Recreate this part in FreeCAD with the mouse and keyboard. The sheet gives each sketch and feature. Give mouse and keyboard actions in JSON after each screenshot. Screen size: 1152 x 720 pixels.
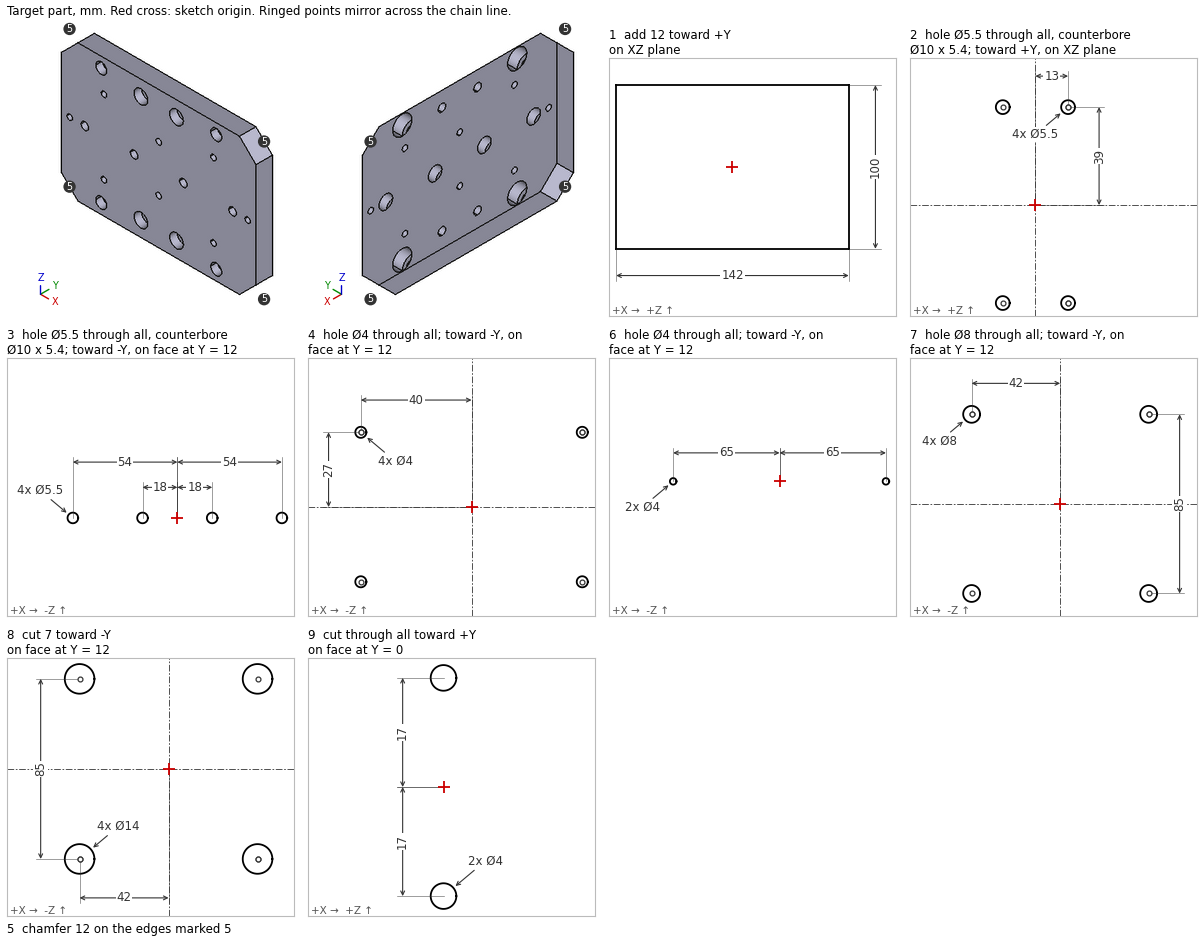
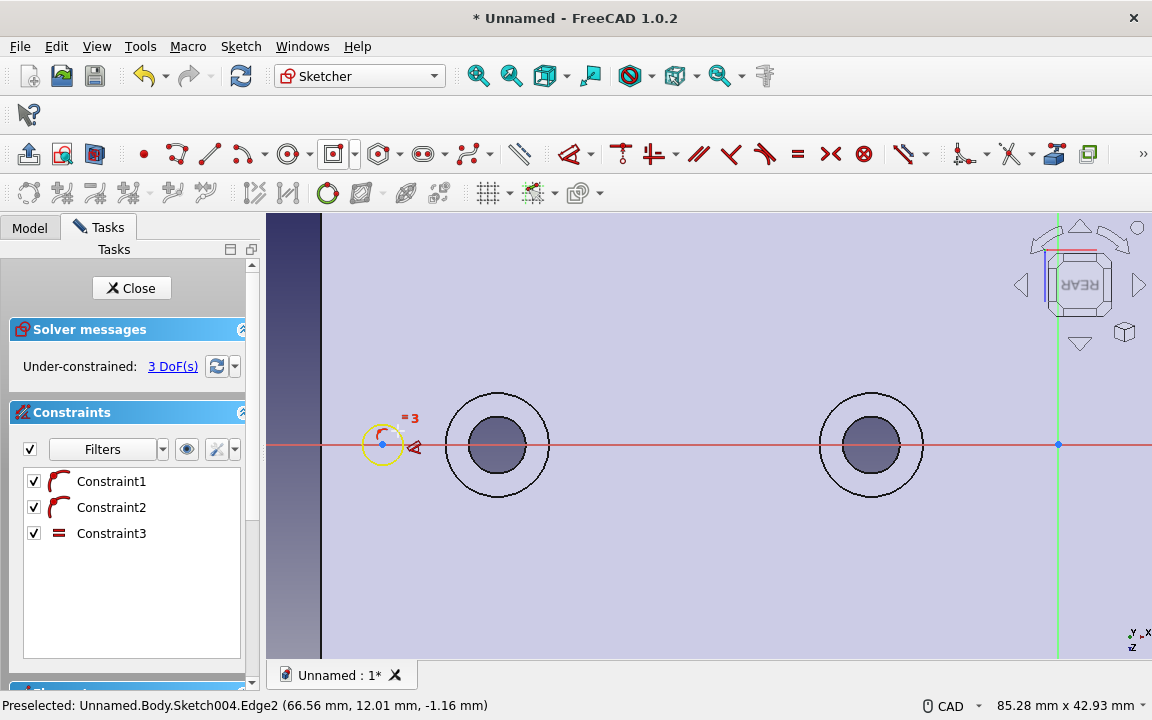
{"action": "left_click", "coordinate": [397, 431]}
{"action": "left_click", "coordinate": [420, 409]}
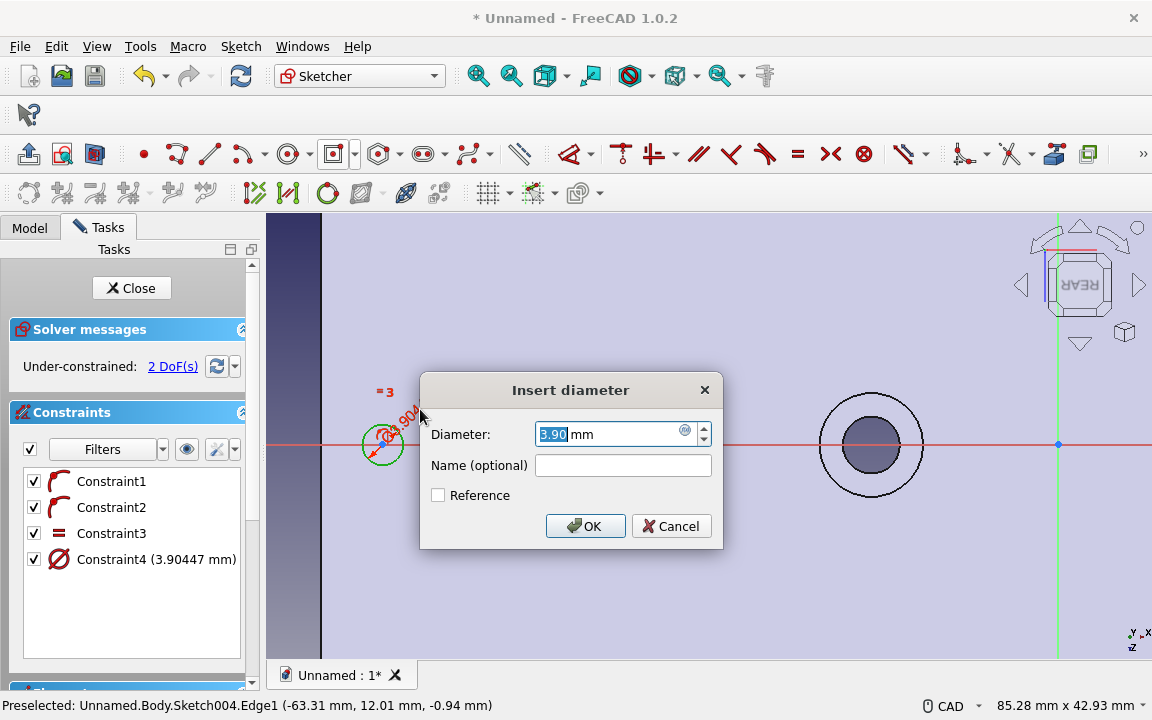
{"action": "type", "text": "4"}
{"action": "key", "text": "Return"}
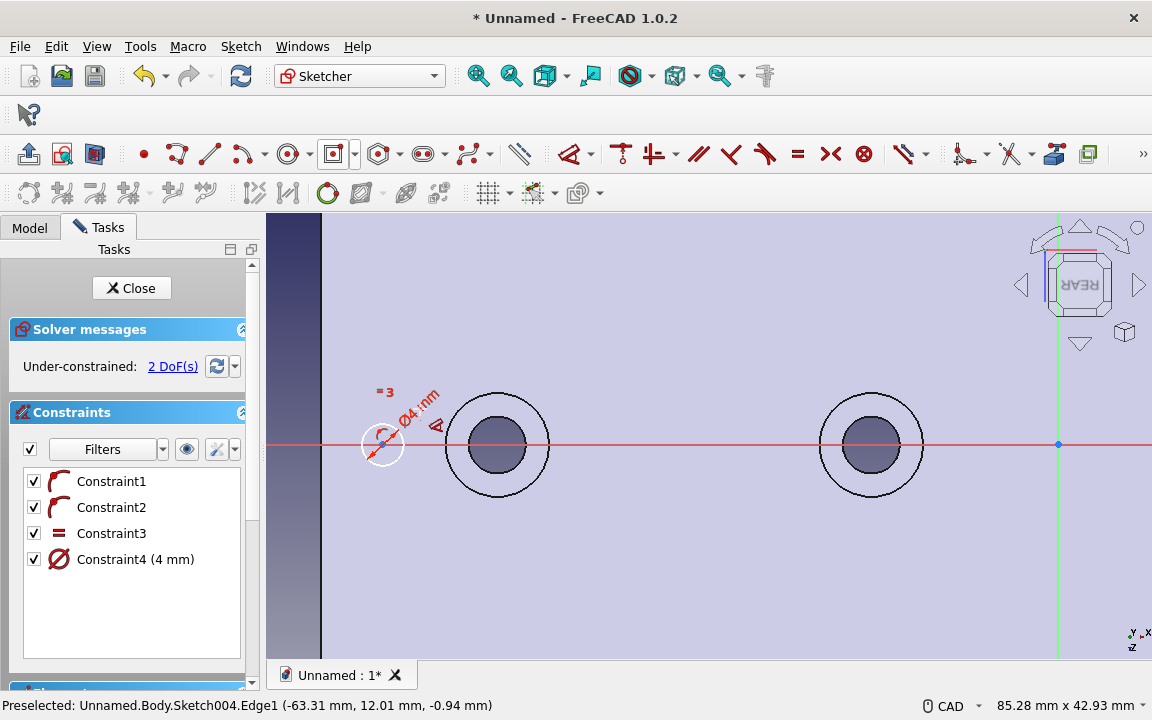
{"action": "left_click", "coordinate": [383, 445]}
{"action": "left_click", "coordinate": [685, 479]}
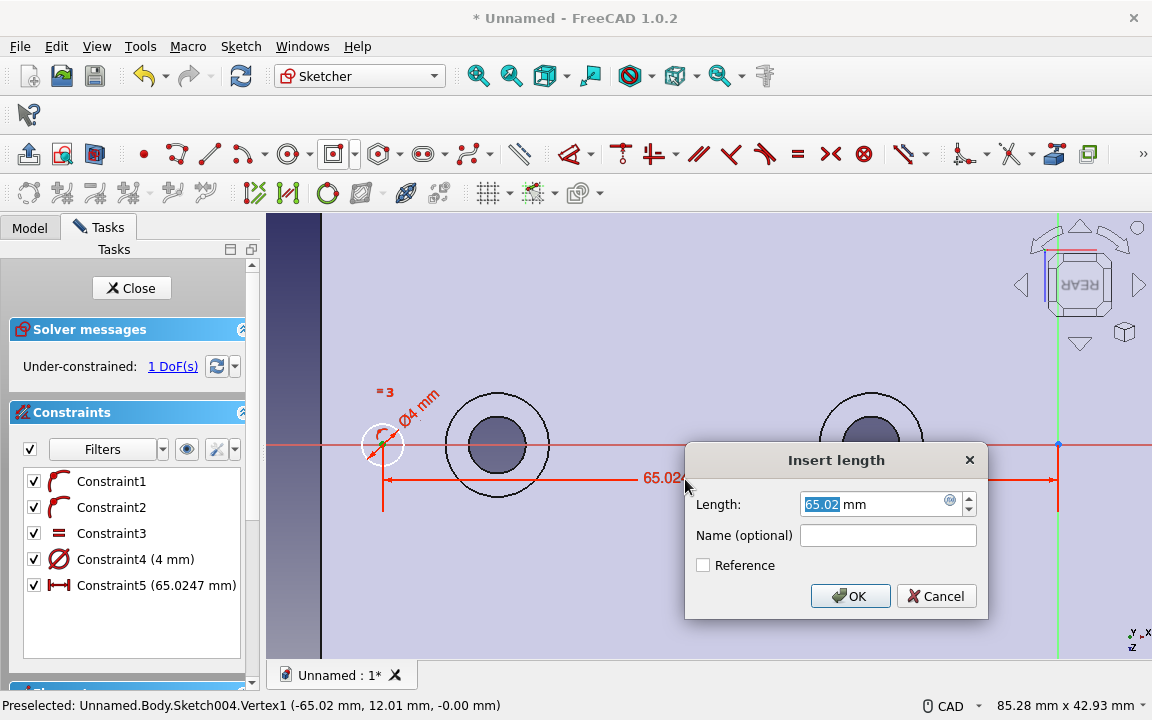
{"action": "type", "text": "65"}
{"action": "key", "text": "Return"}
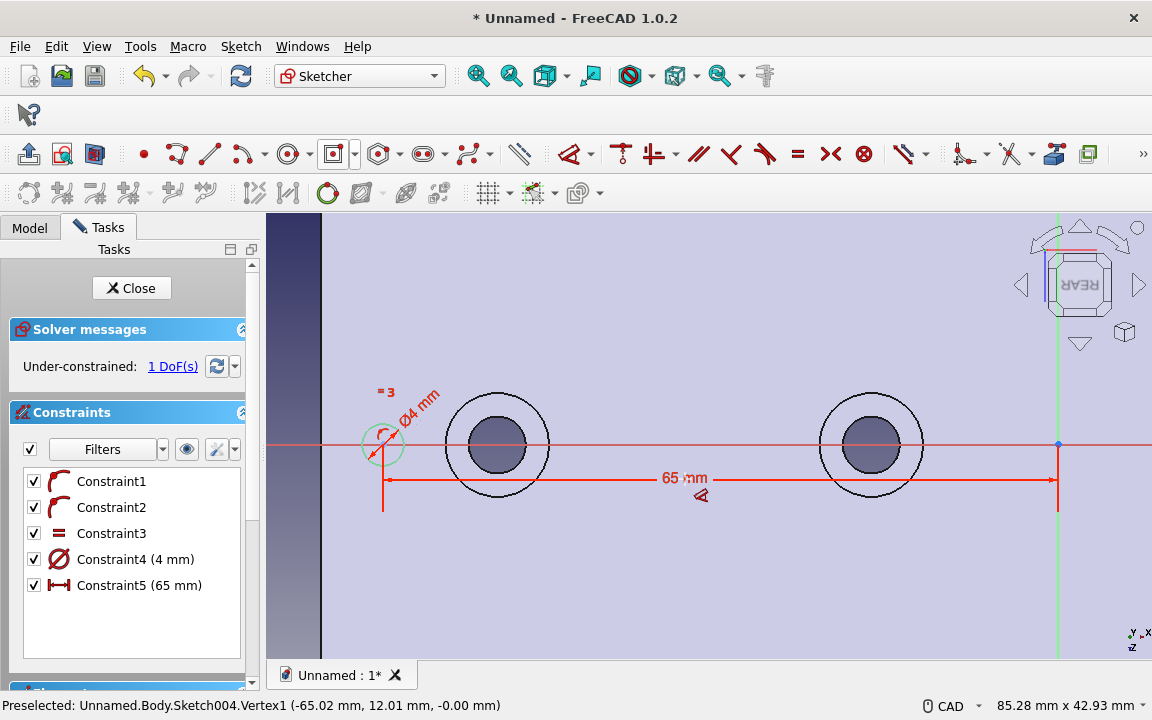
{"action": "scroll", "coordinate": [397, 431], "scroll_direction": "down", "scroll_amount": 5}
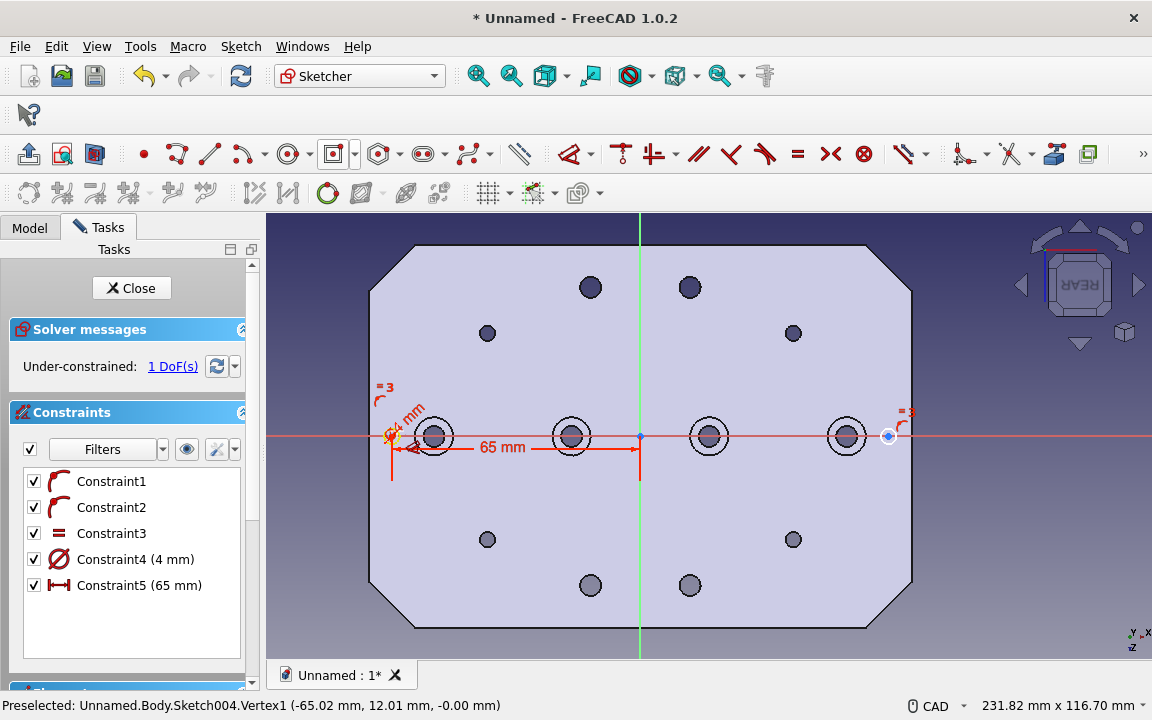
{"action": "left_click", "coordinate": [889, 436]}
{"action": "left_click", "coordinate": [765, 470]}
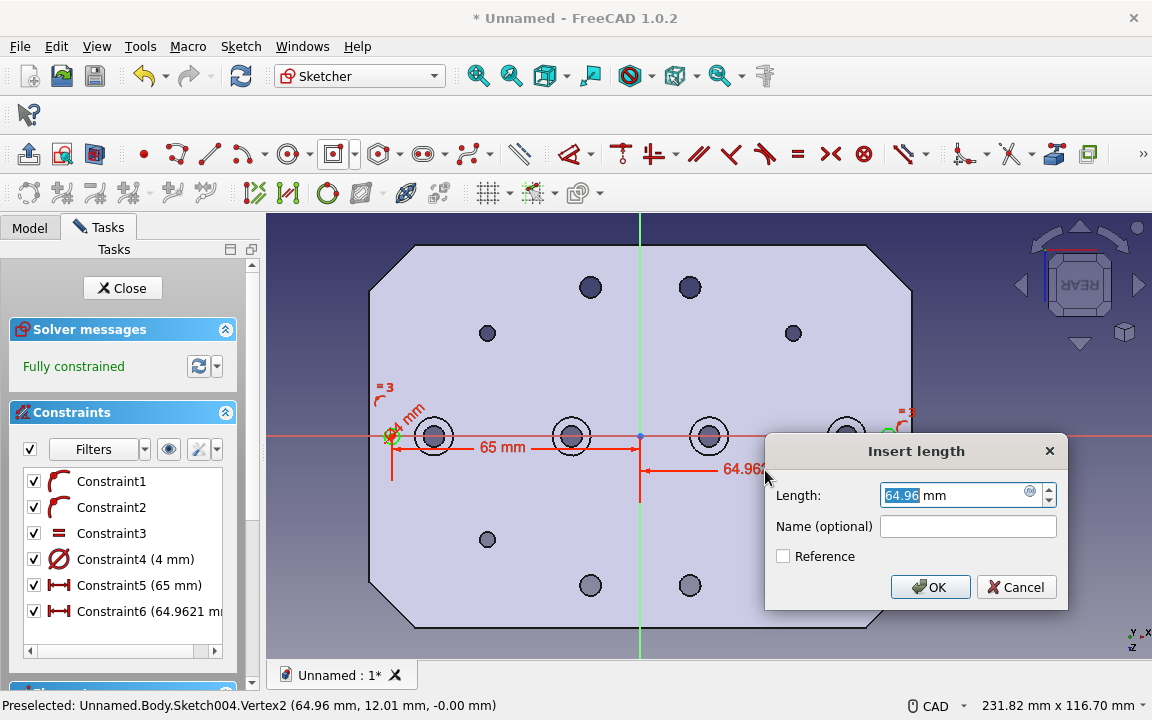
{"action": "type", "text": "65"}
{"action": "key", "text": "Return"}
{"action": "key", "text": "Escape"}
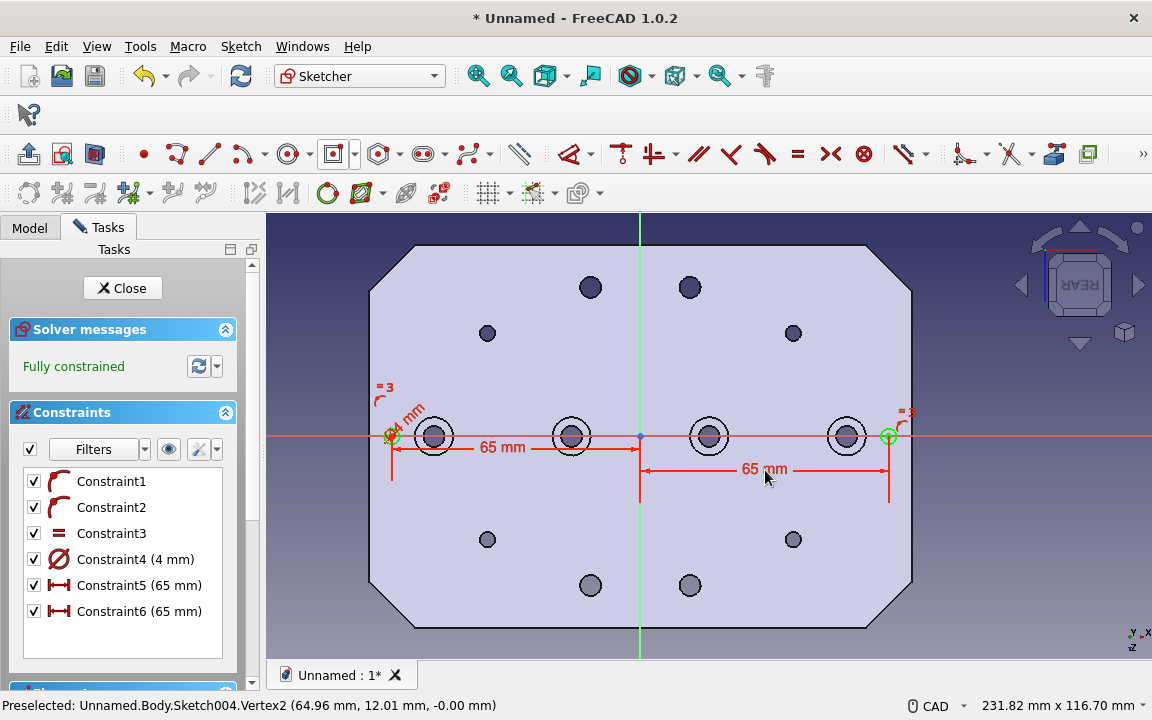
{"action": "left_click", "coordinate": [123, 288]}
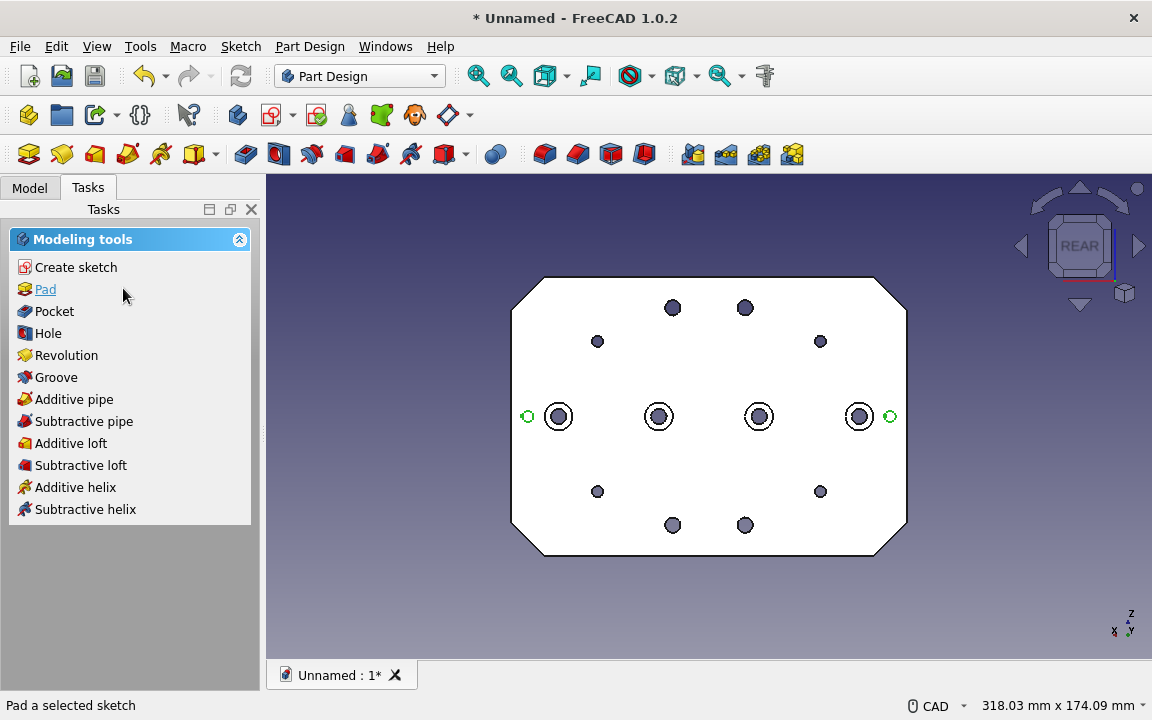
{"action": "left_click", "coordinate": [279, 154]}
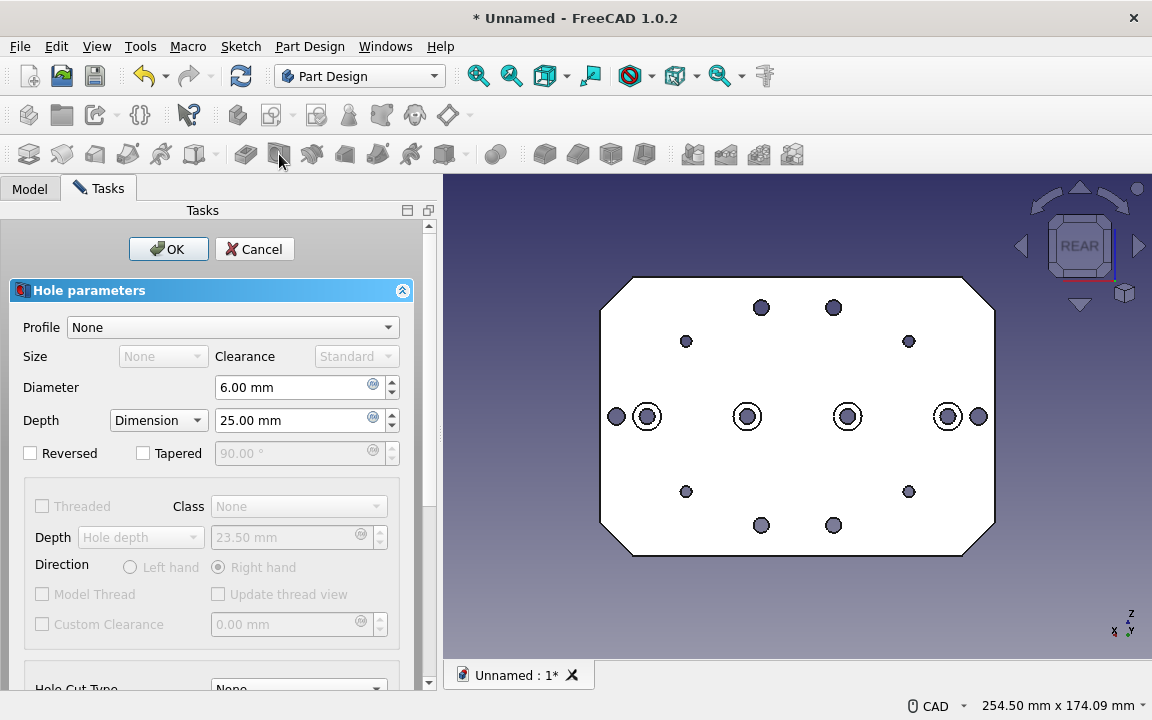
{"action": "triple_click", "coordinate": [300, 388]}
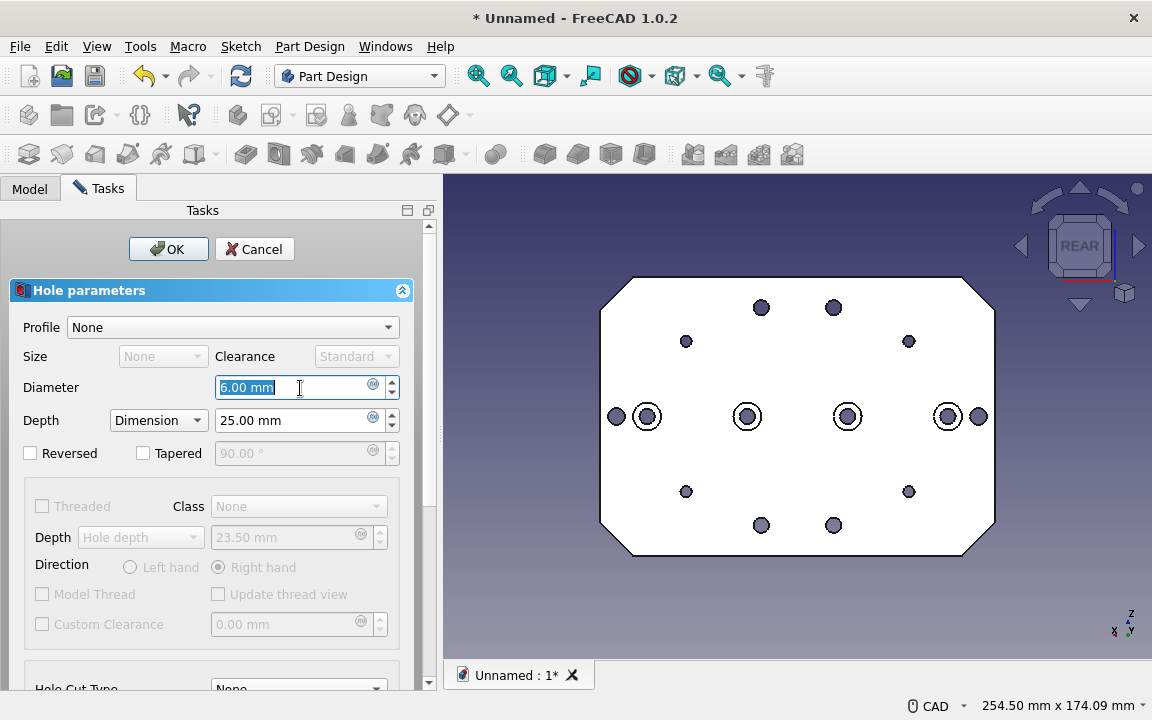
{"action": "type", "text": "4"}
{"action": "key", "text": "Tab"}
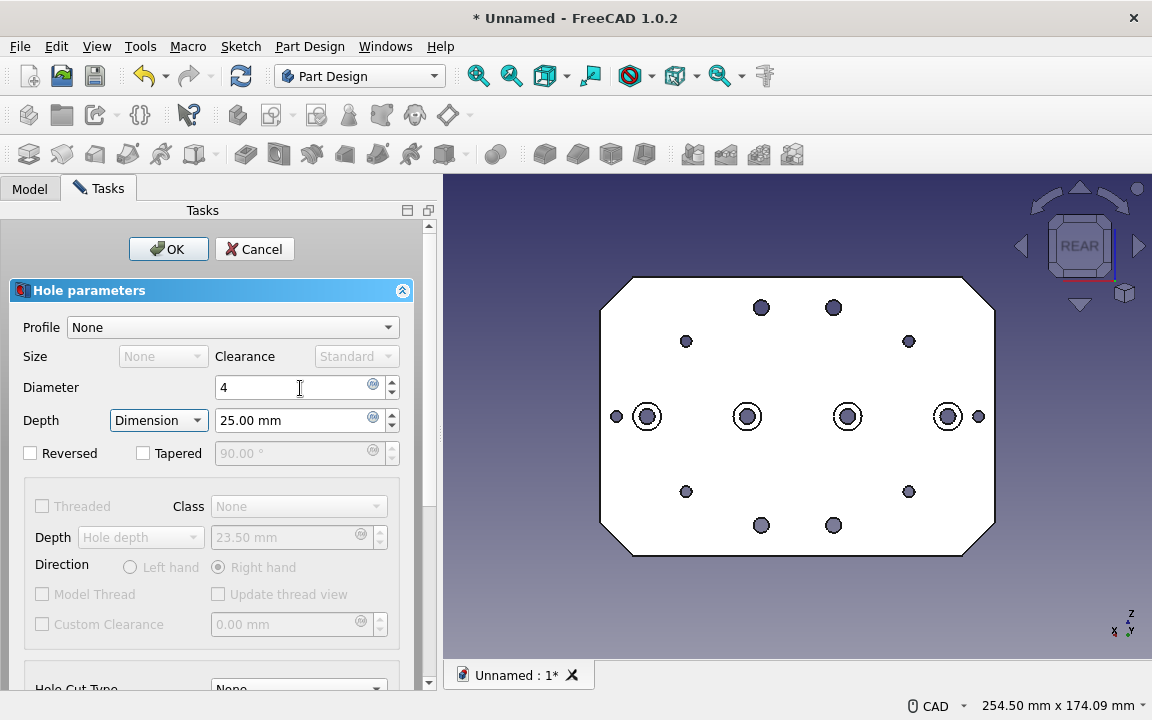
{"action": "left_click", "coordinate": [160, 420]}